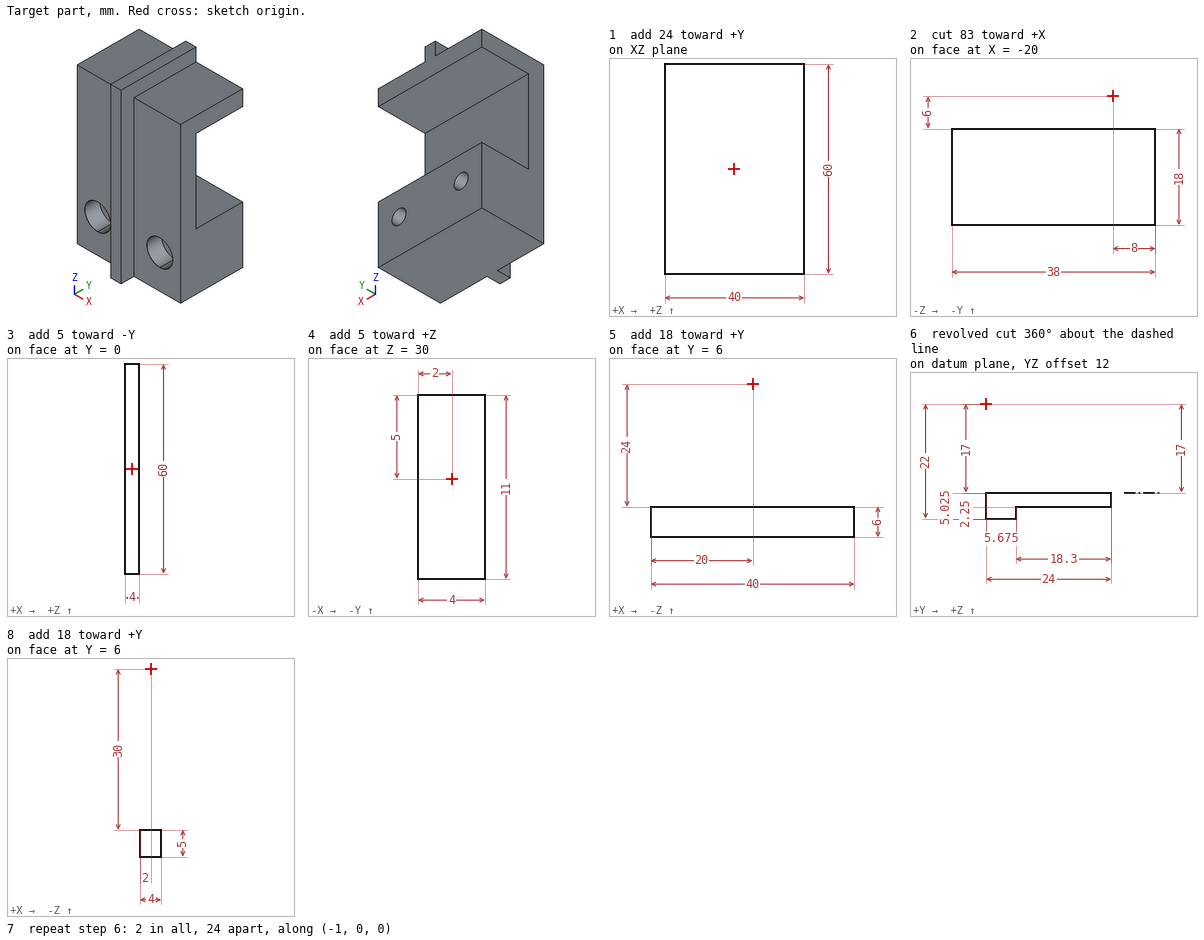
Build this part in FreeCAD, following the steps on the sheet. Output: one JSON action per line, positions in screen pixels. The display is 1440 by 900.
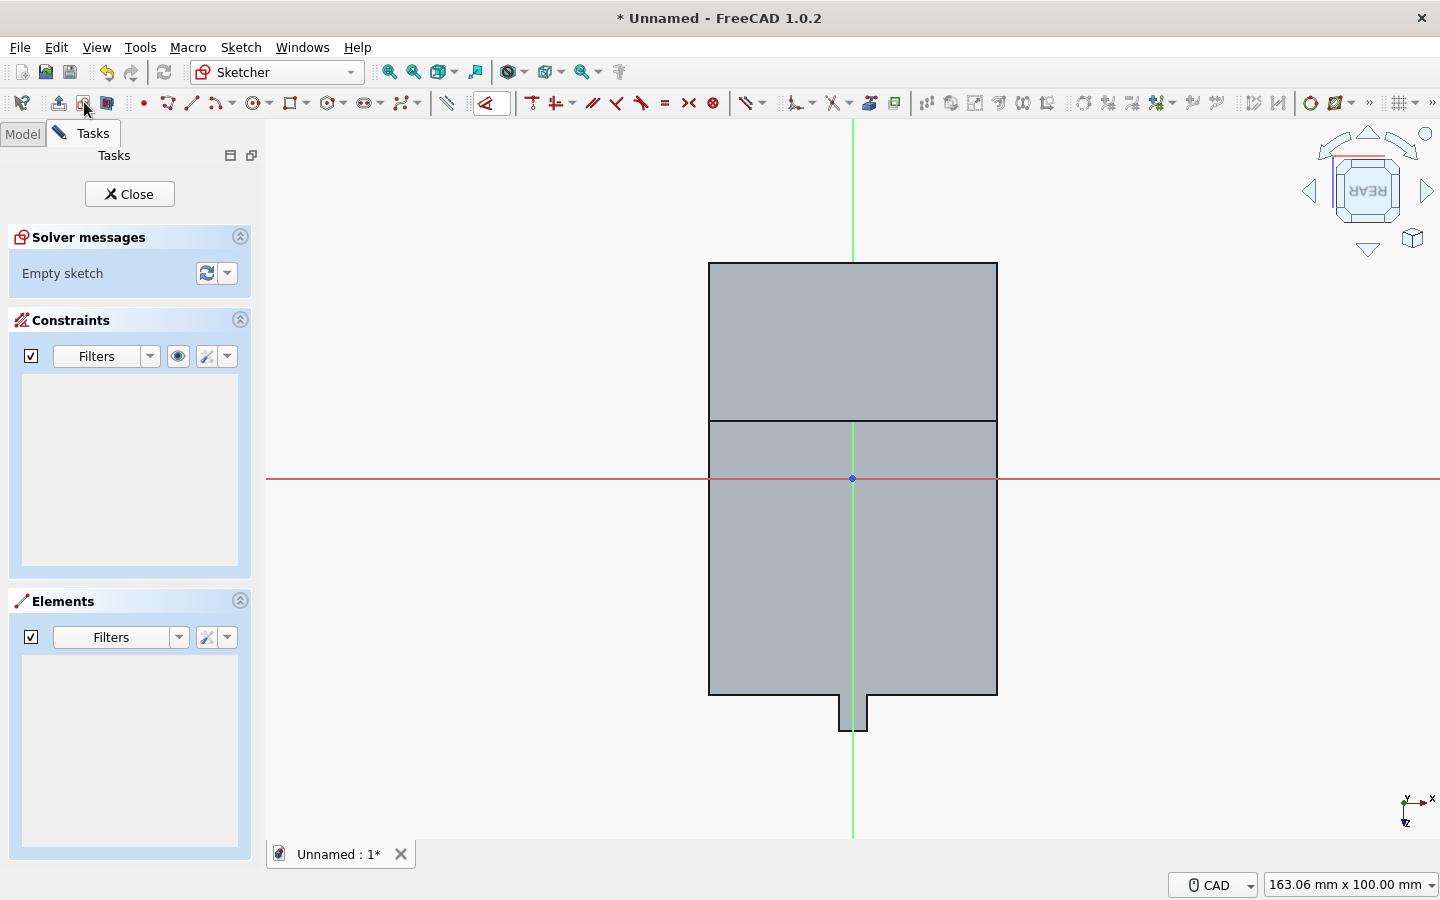
{"action": "scroll", "coordinate": [909, 675], "scroll_direction": "up", "scroll_amount": 4}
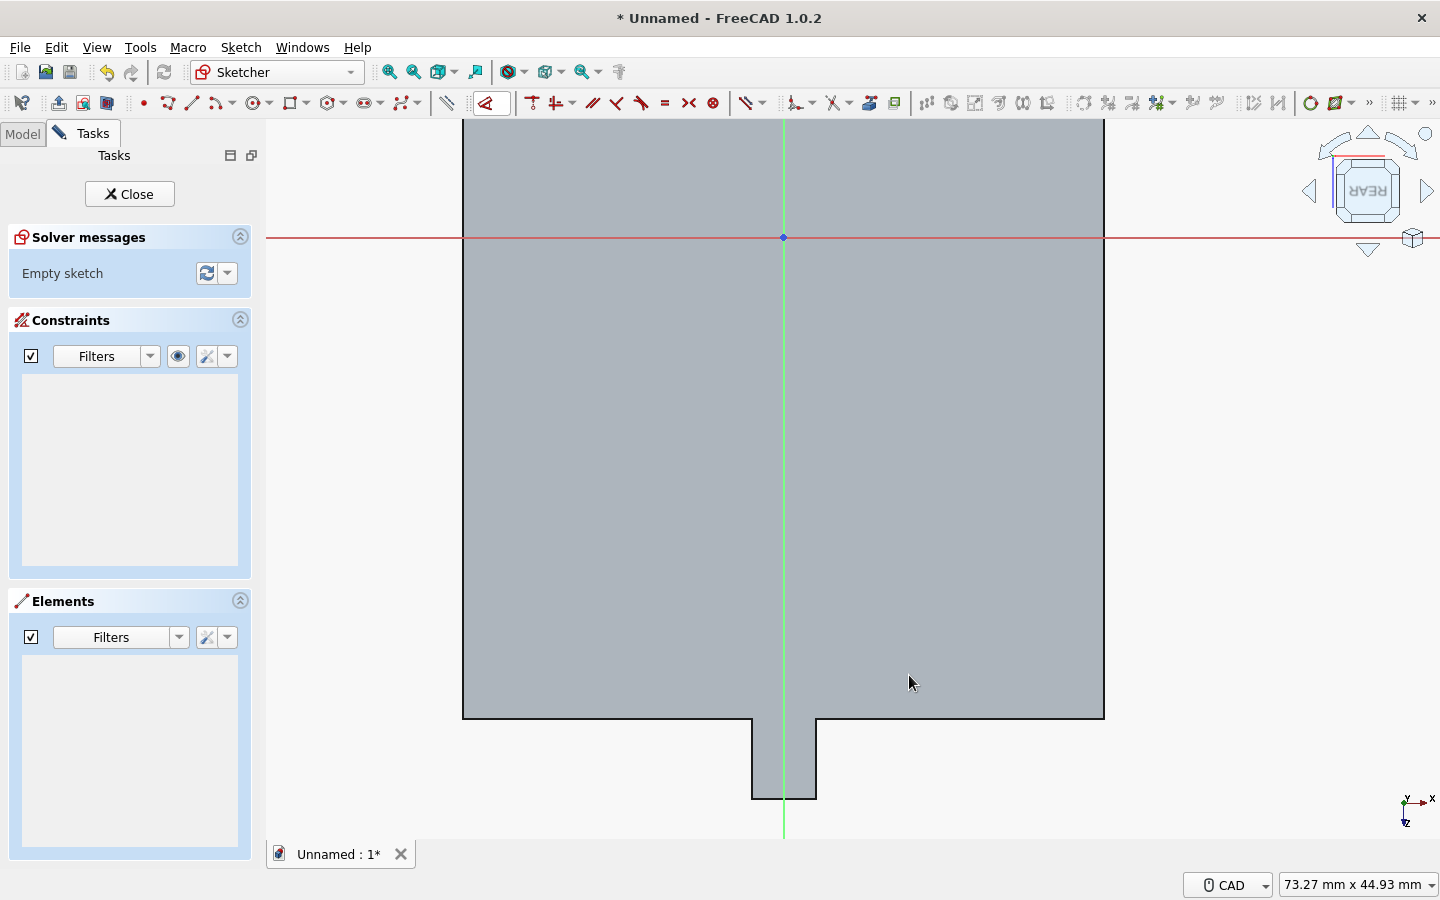
{"action": "key", "text": "g r"}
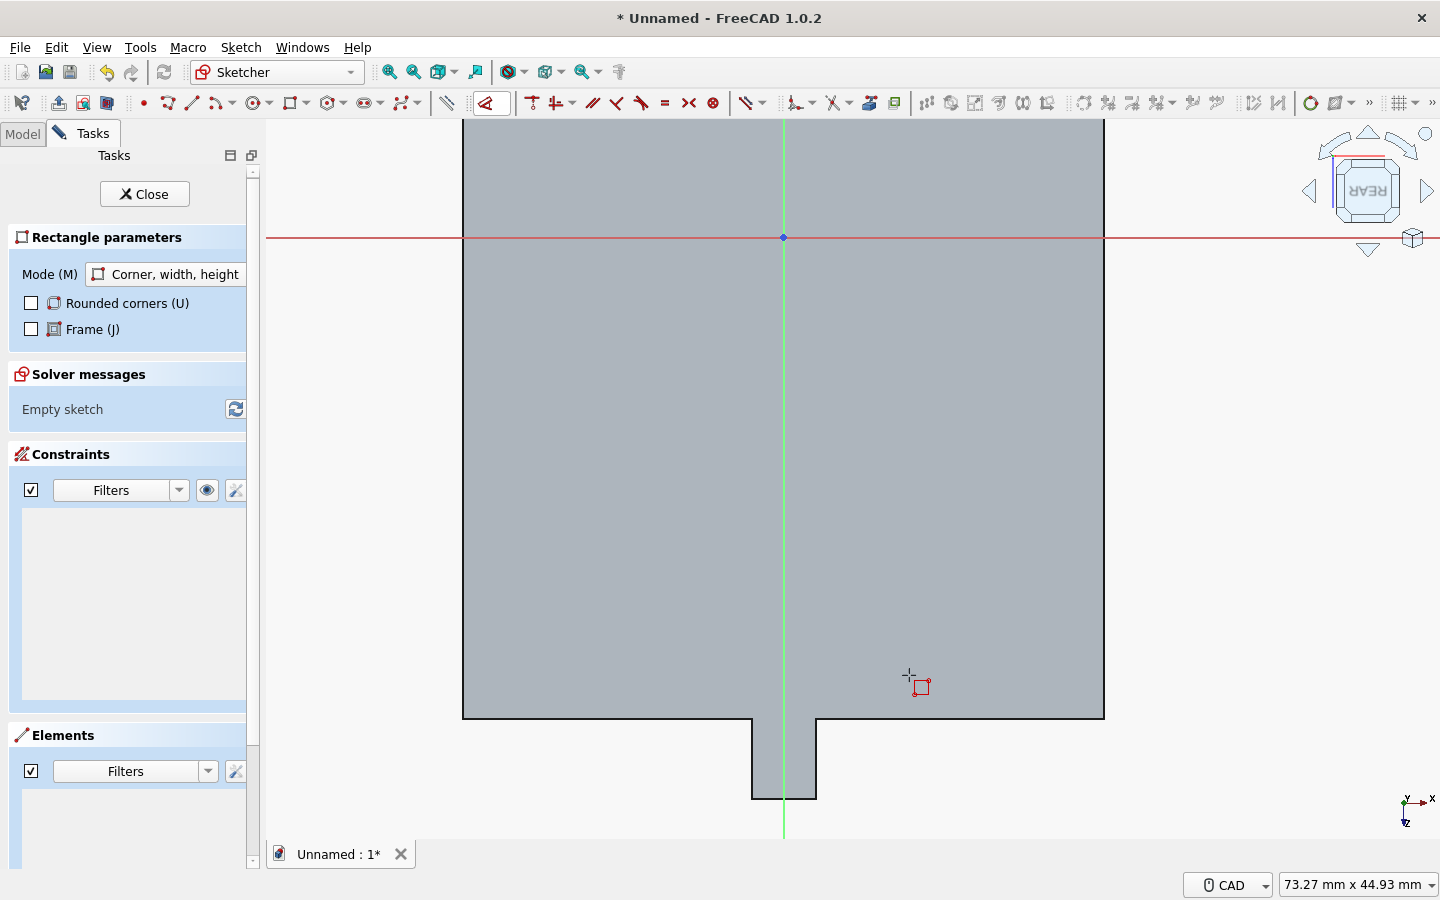
{"action": "left_click", "coordinate": [463, 622]}
{"action": "mouse_move", "coordinate": [1104, 719]}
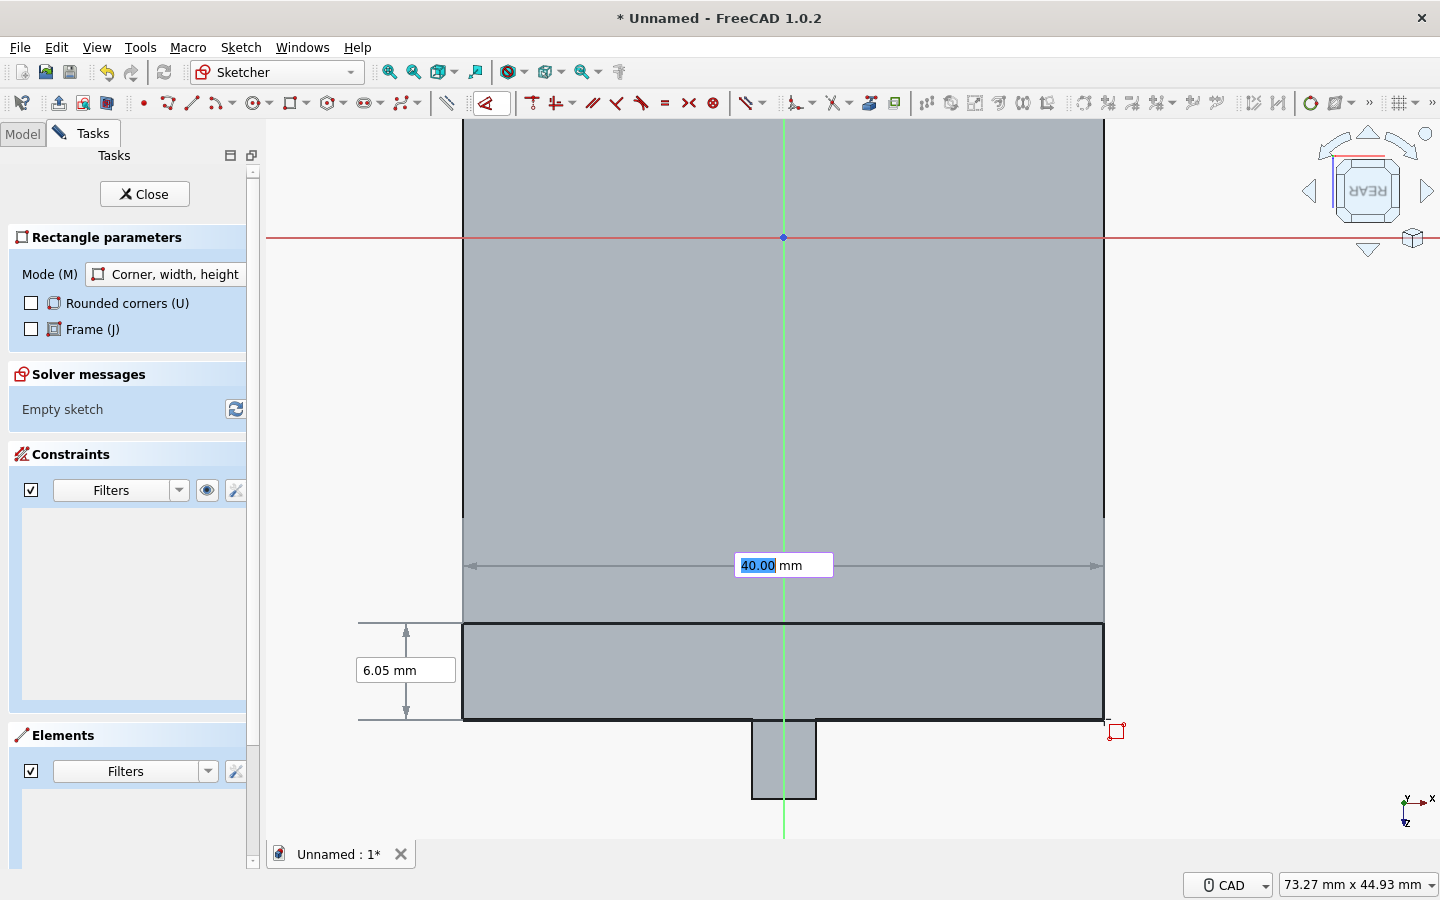
{"action": "type", "text": "40"}
{"action": "key", "text": "Tab"}
{"action": "type", "text": "6"}
{"action": "key", "text": "Return"}
{"action": "key", "text": "Escape"}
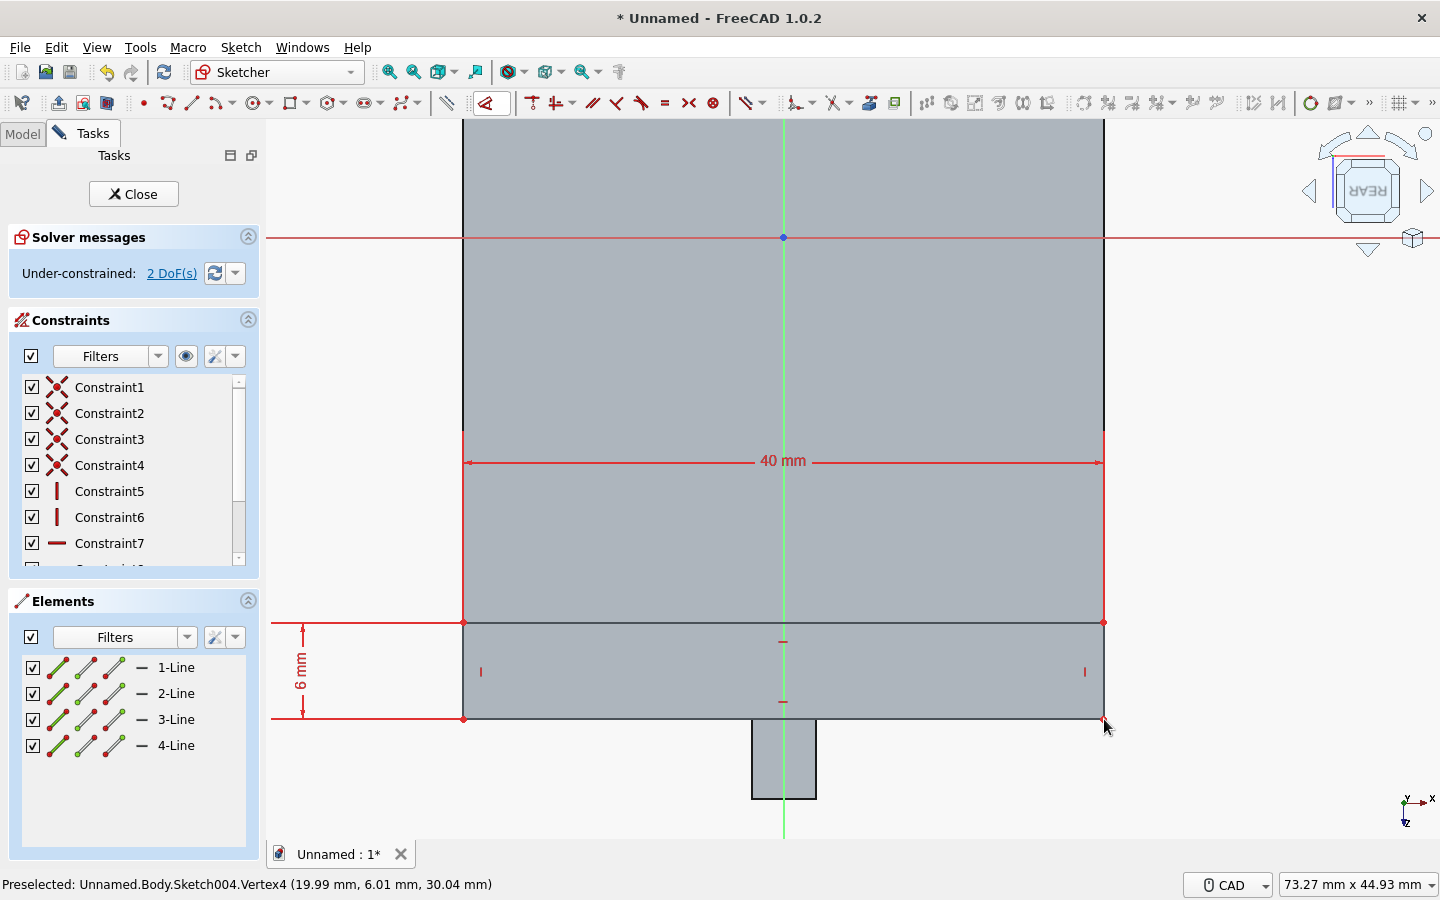
{"action": "key", "text": "d"}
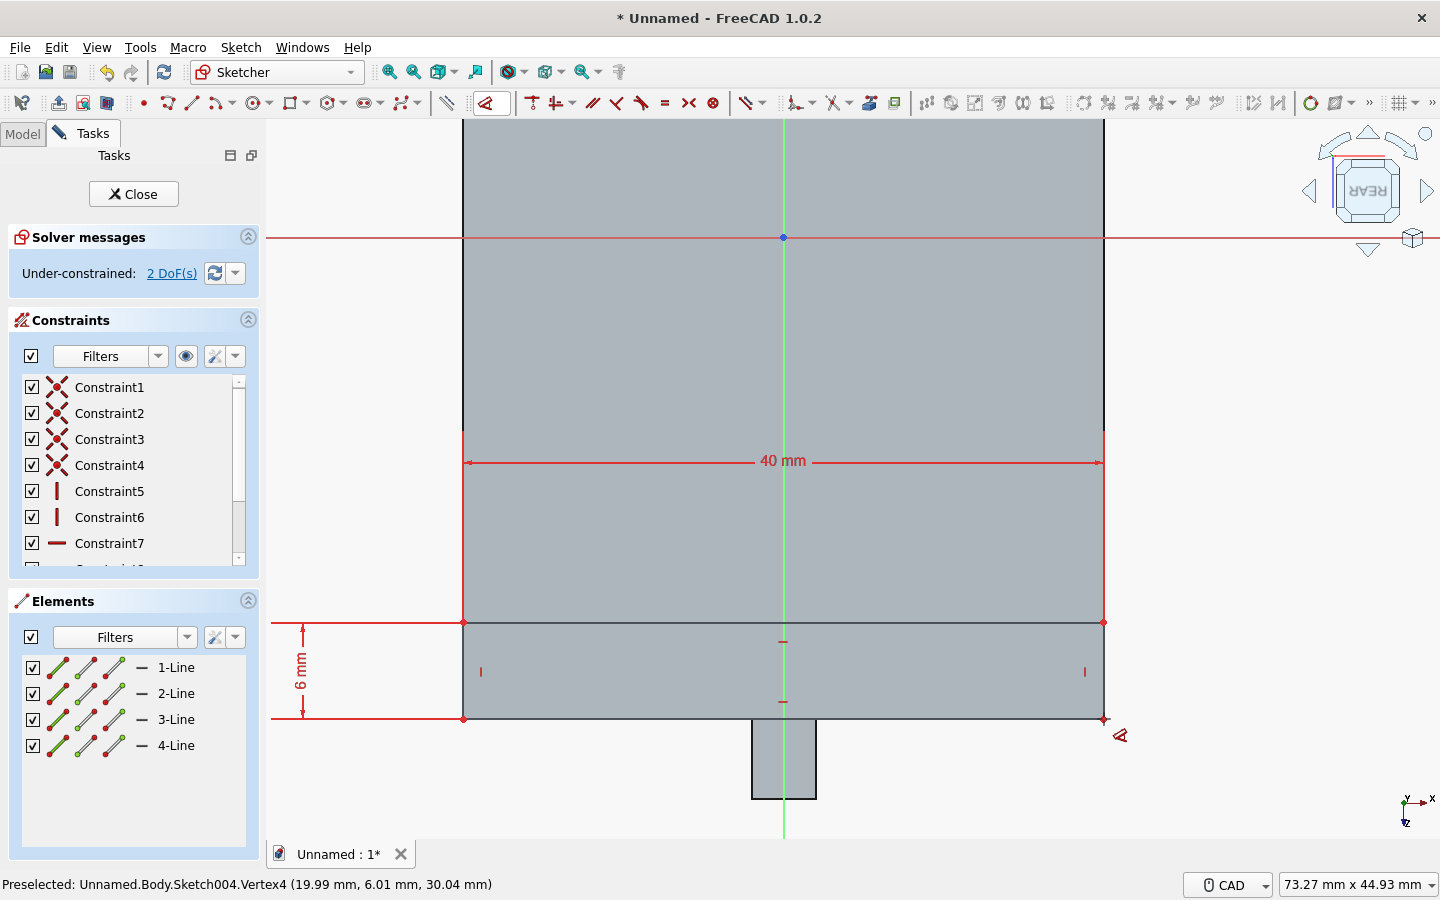
{"action": "left_click", "coordinate": [463, 623]}
{"action": "left_click", "coordinate": [623, 204]}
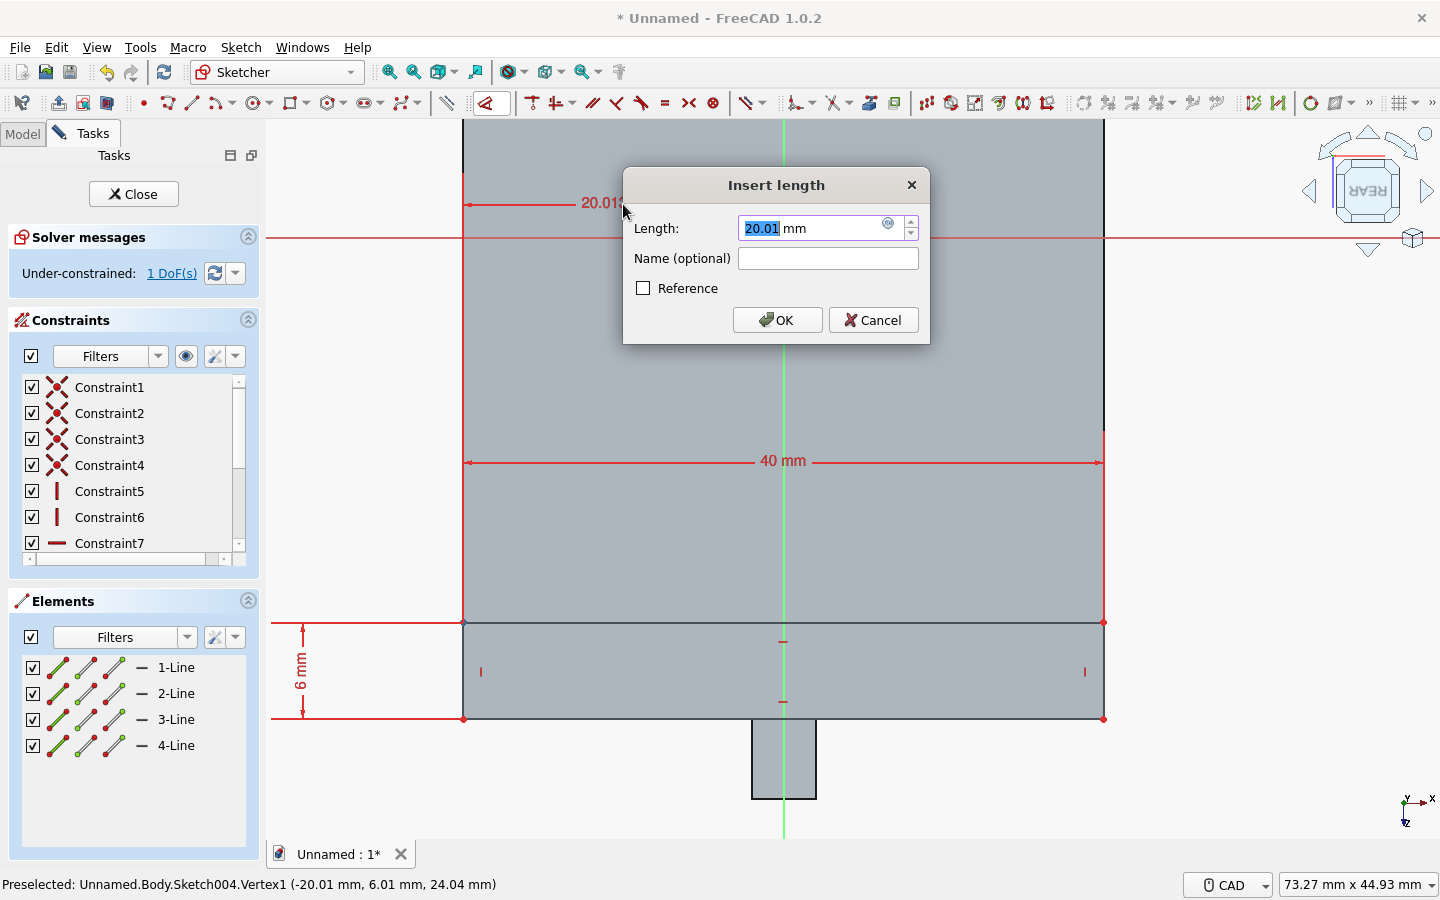
{"action": "type", "text": "20"}
{"action": "key", "text": "Return"}